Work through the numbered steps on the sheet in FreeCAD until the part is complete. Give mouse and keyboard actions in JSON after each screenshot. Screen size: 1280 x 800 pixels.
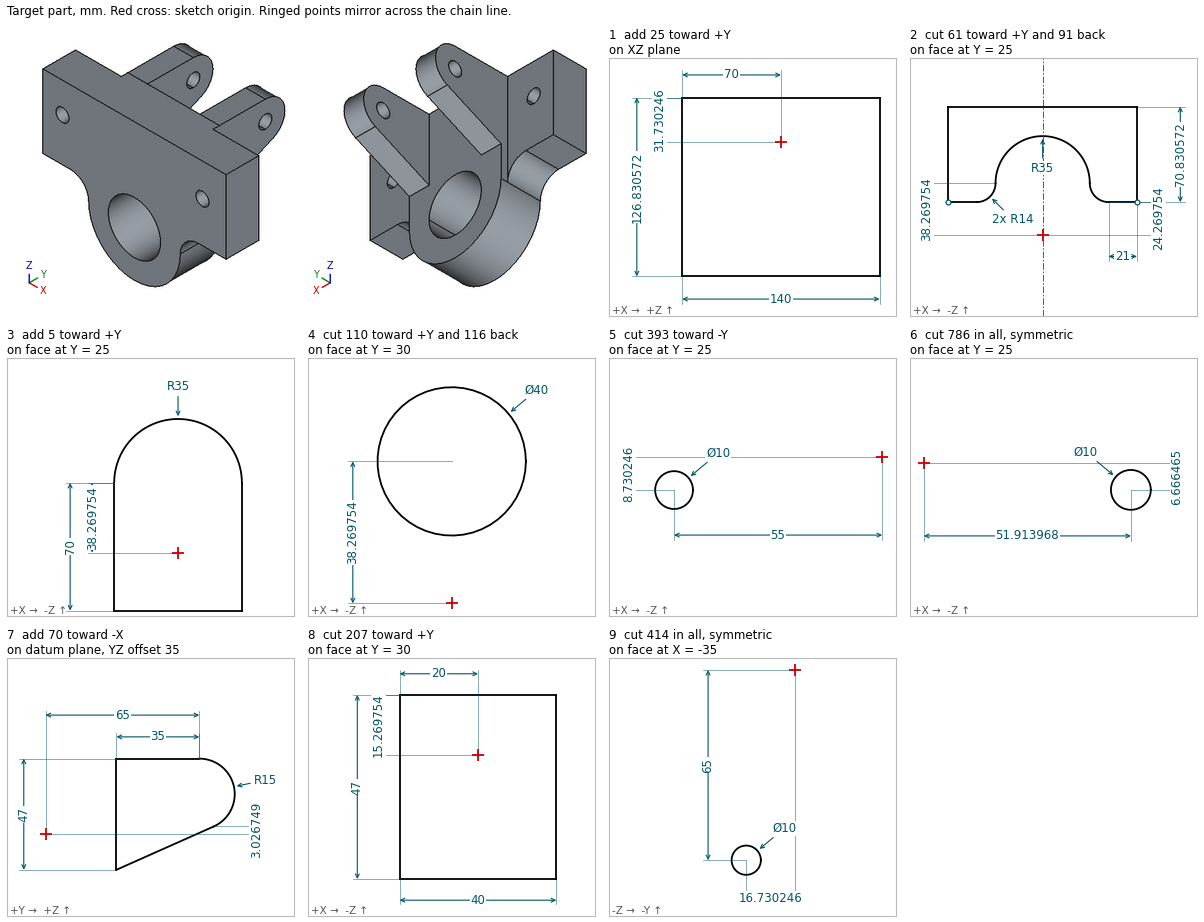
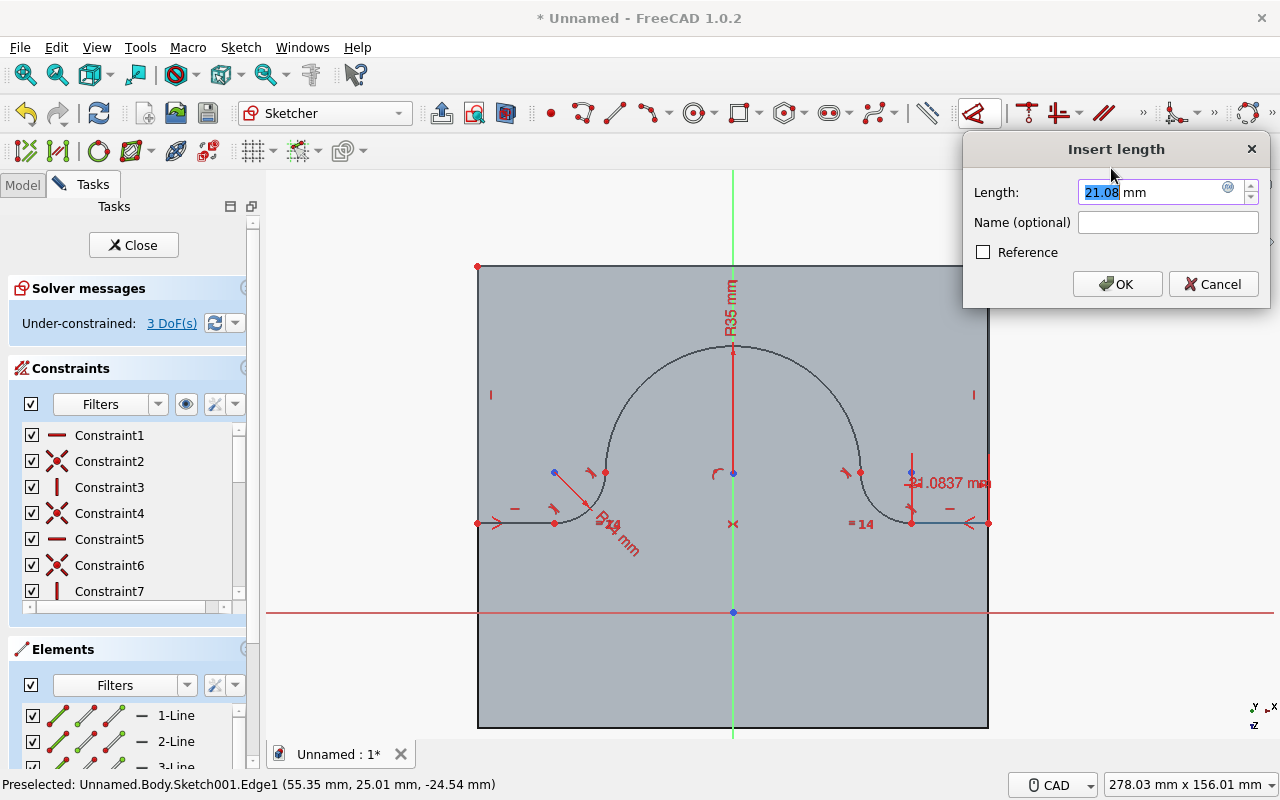
{"action": "type", "text": "21"}
{"action": "key", "text": "Return"}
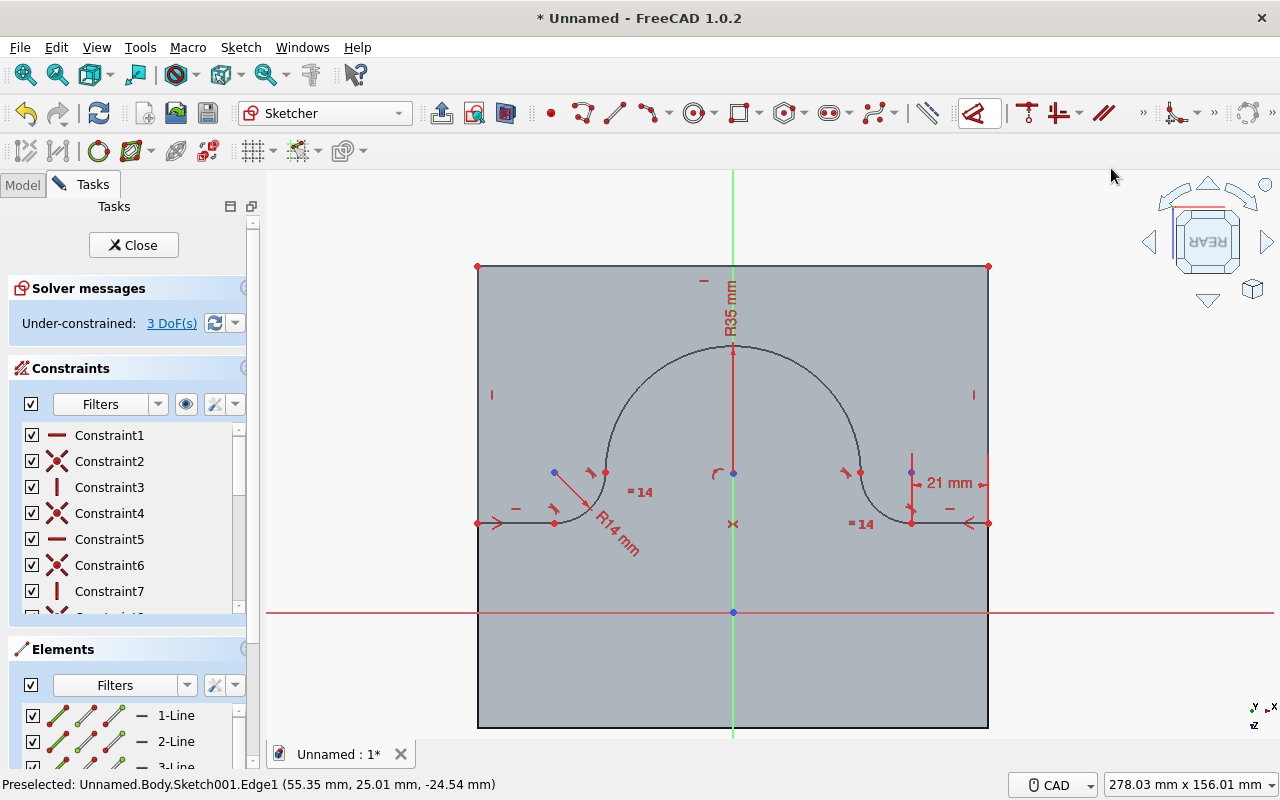
{"action": "left_click", "coordinate": [988, 446]}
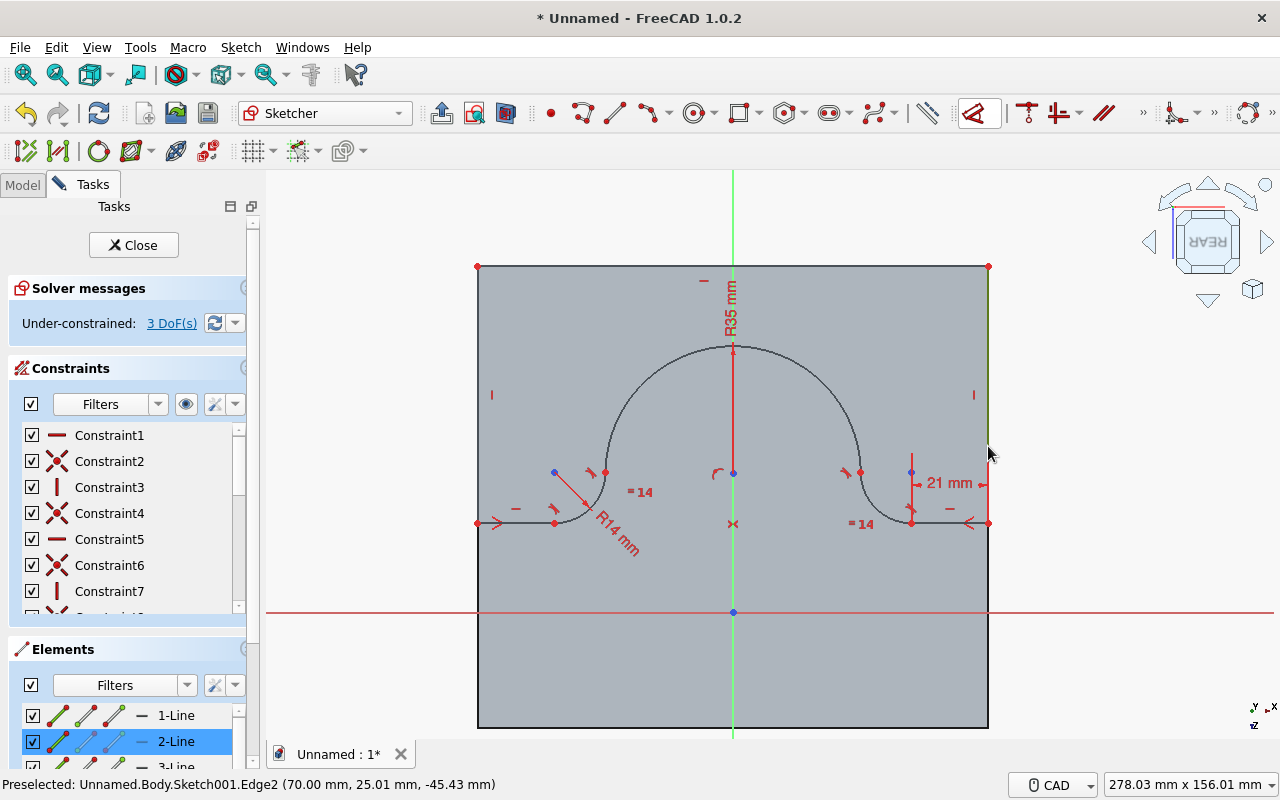
{"action": "key", "text": "i"}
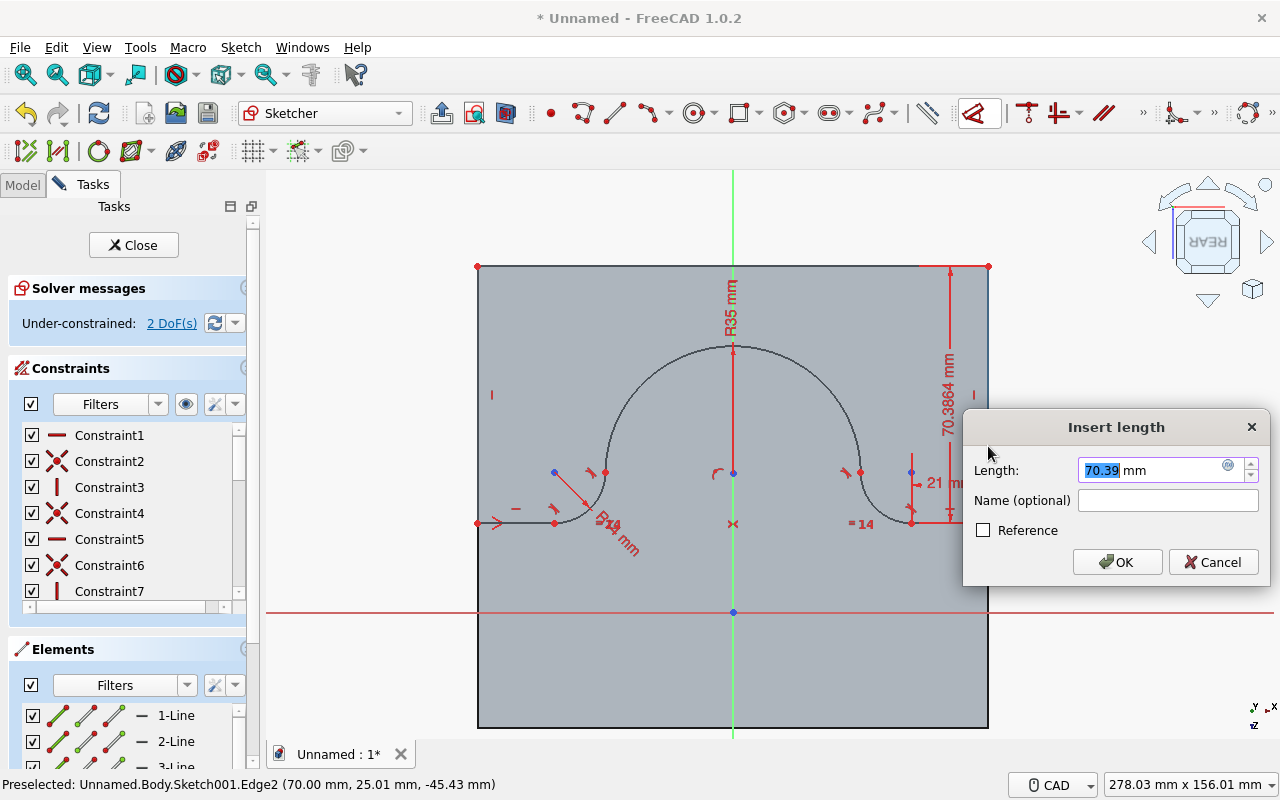
{"action": "type", "text": "70.830572"}
{"action": "key", "text": "Return"}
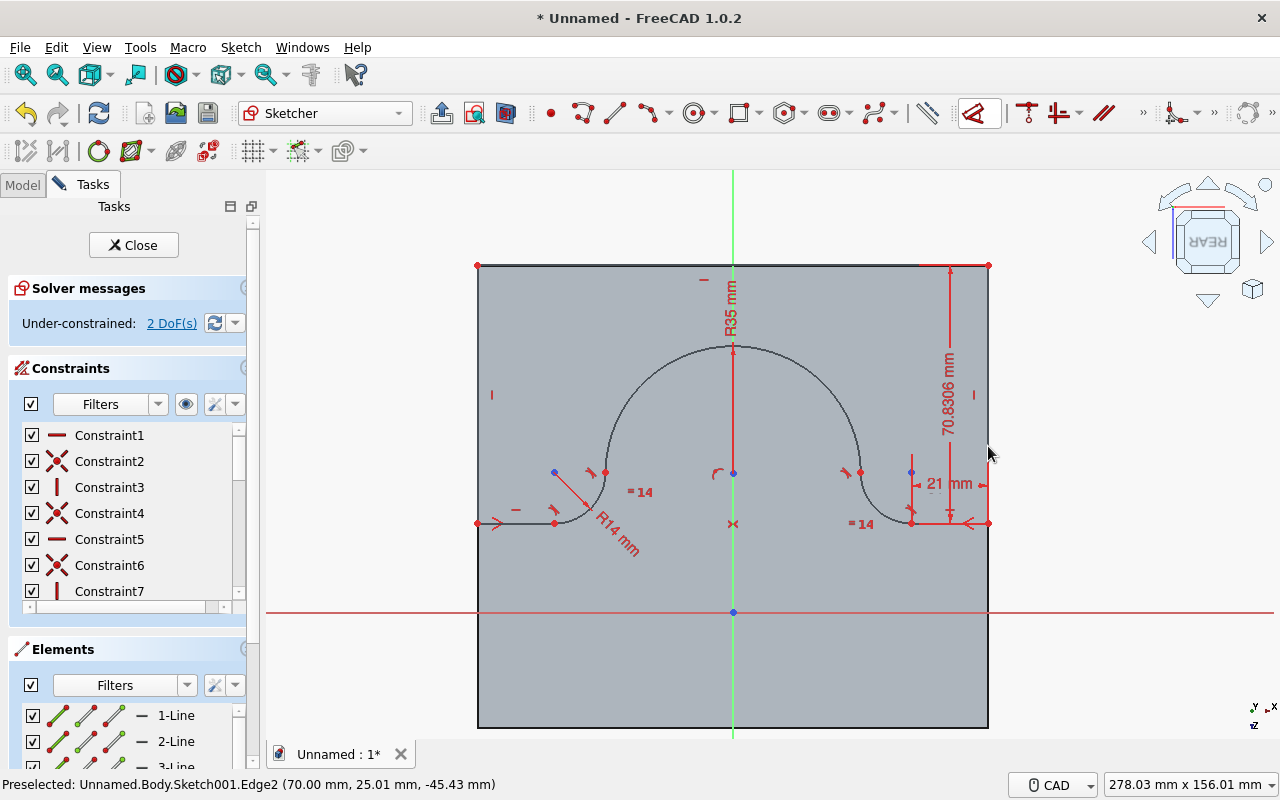
{"action": "left_click", "coordinate": [912, 524]}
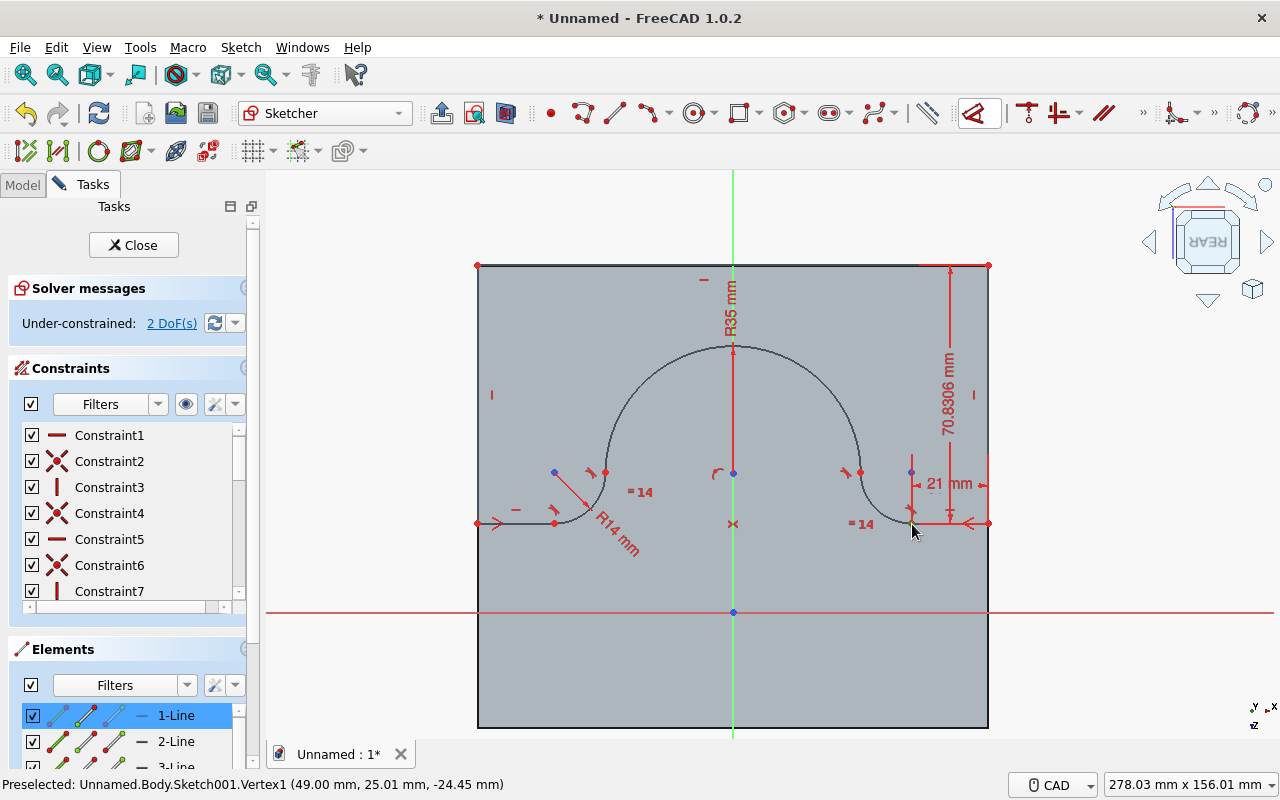
{"action": "key", "text": "i"}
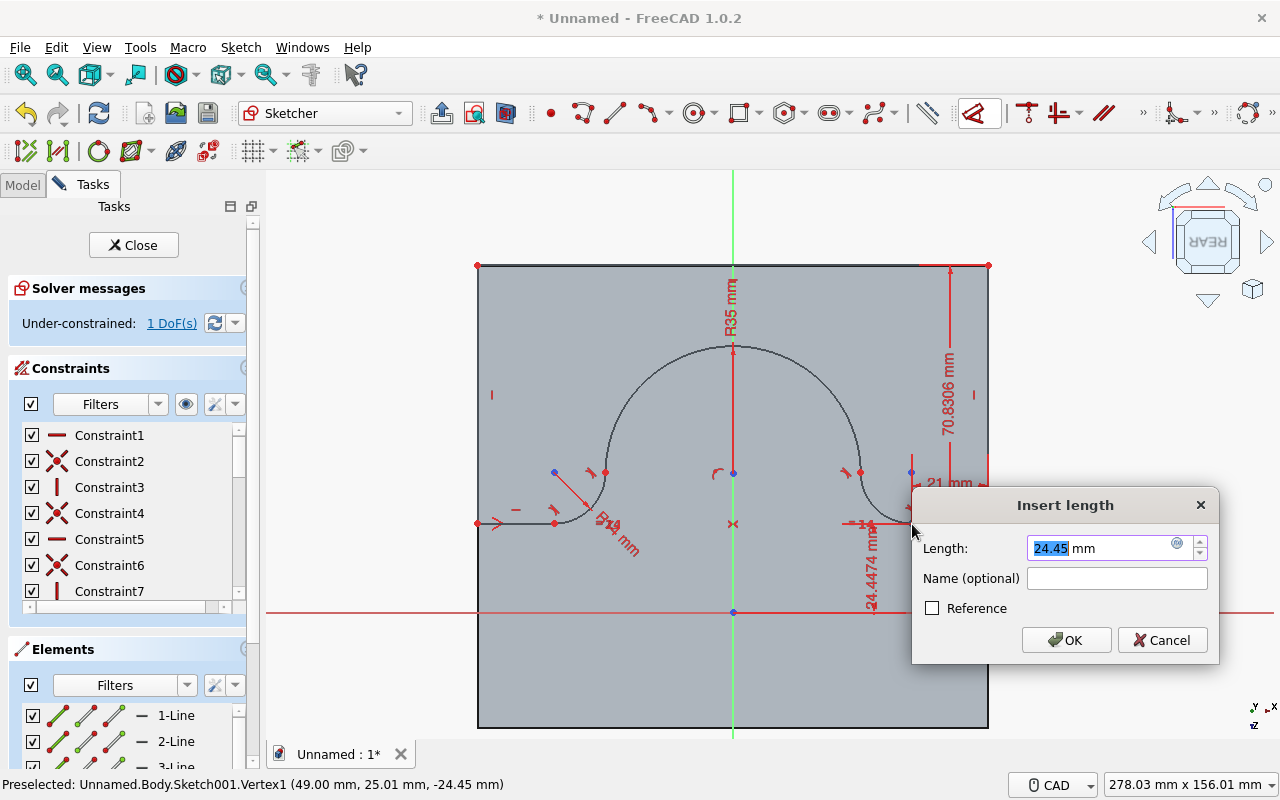
{"action": "type", "text": "24.269754"}
{"action": "key", "text": "Return"}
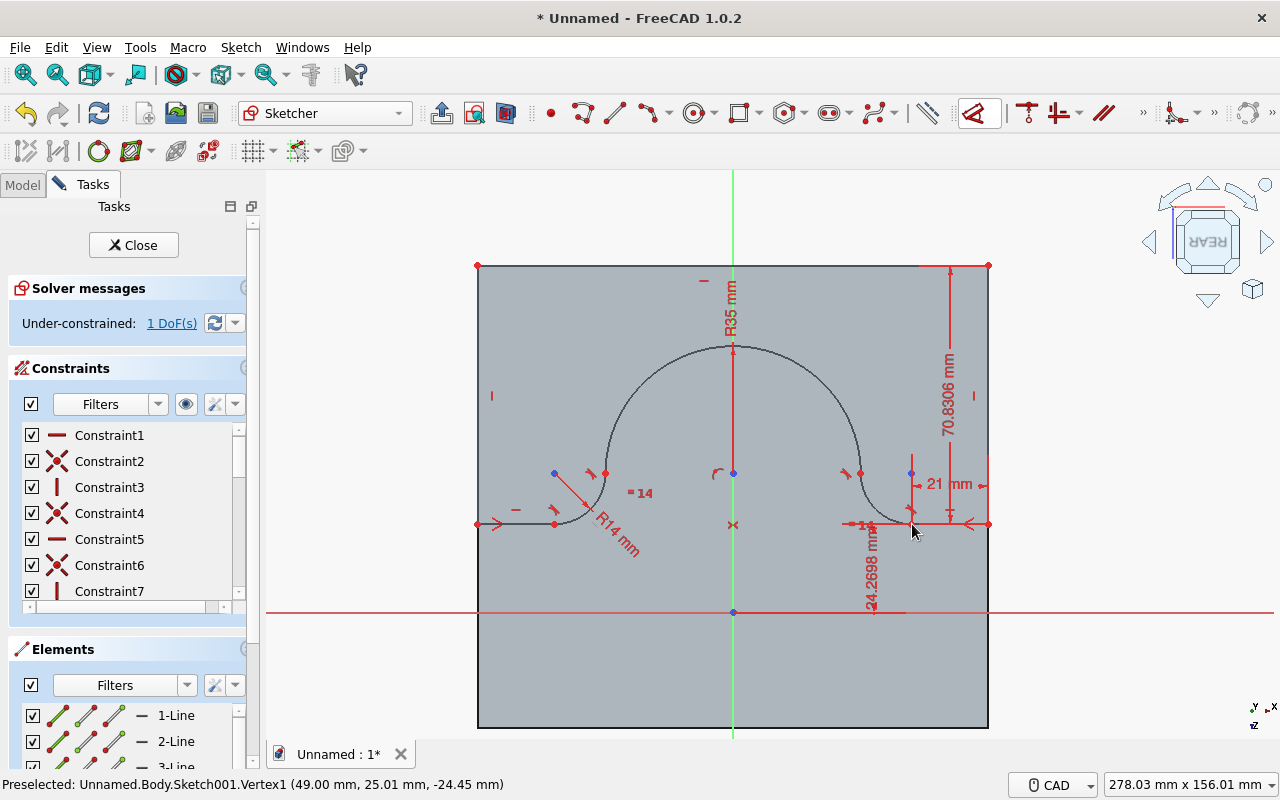
{"action": "left_click", "coordinate": [605, 473]}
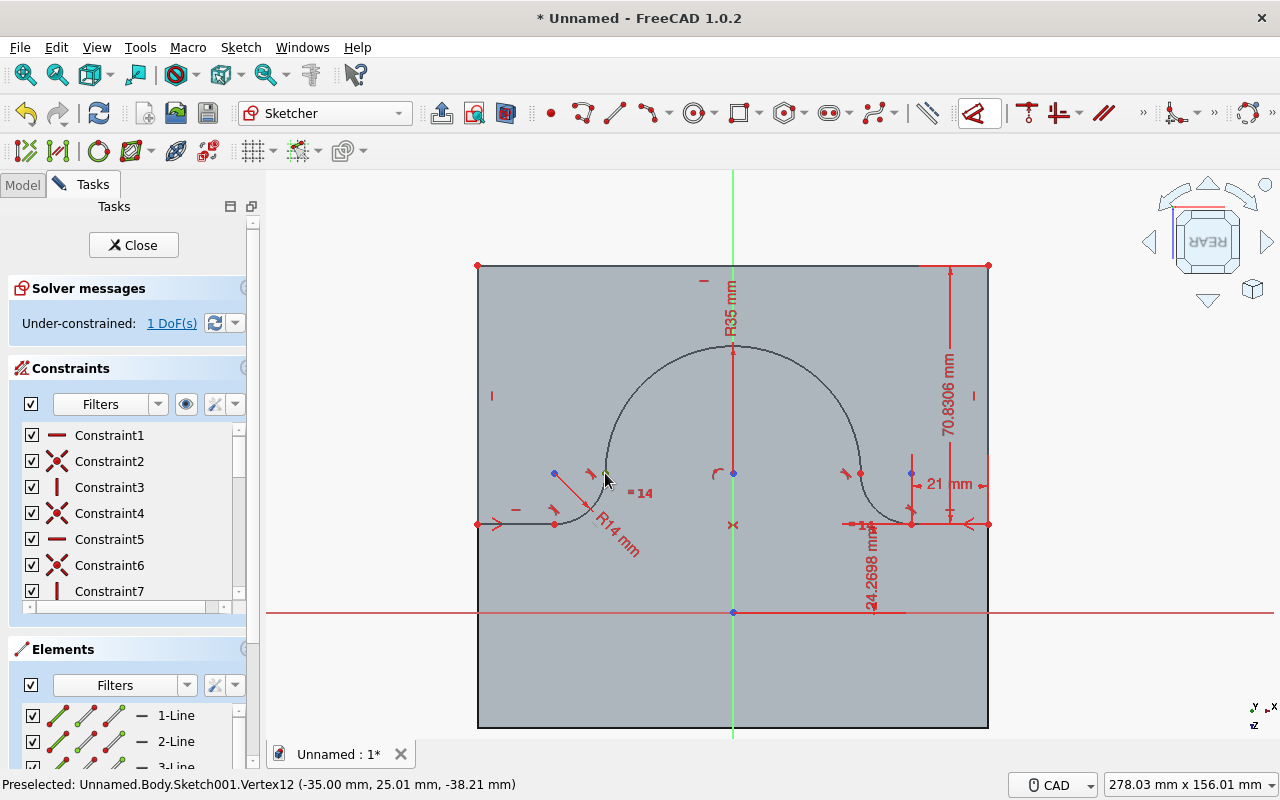
{"action": "left_click", "coordinate": [996, 114]}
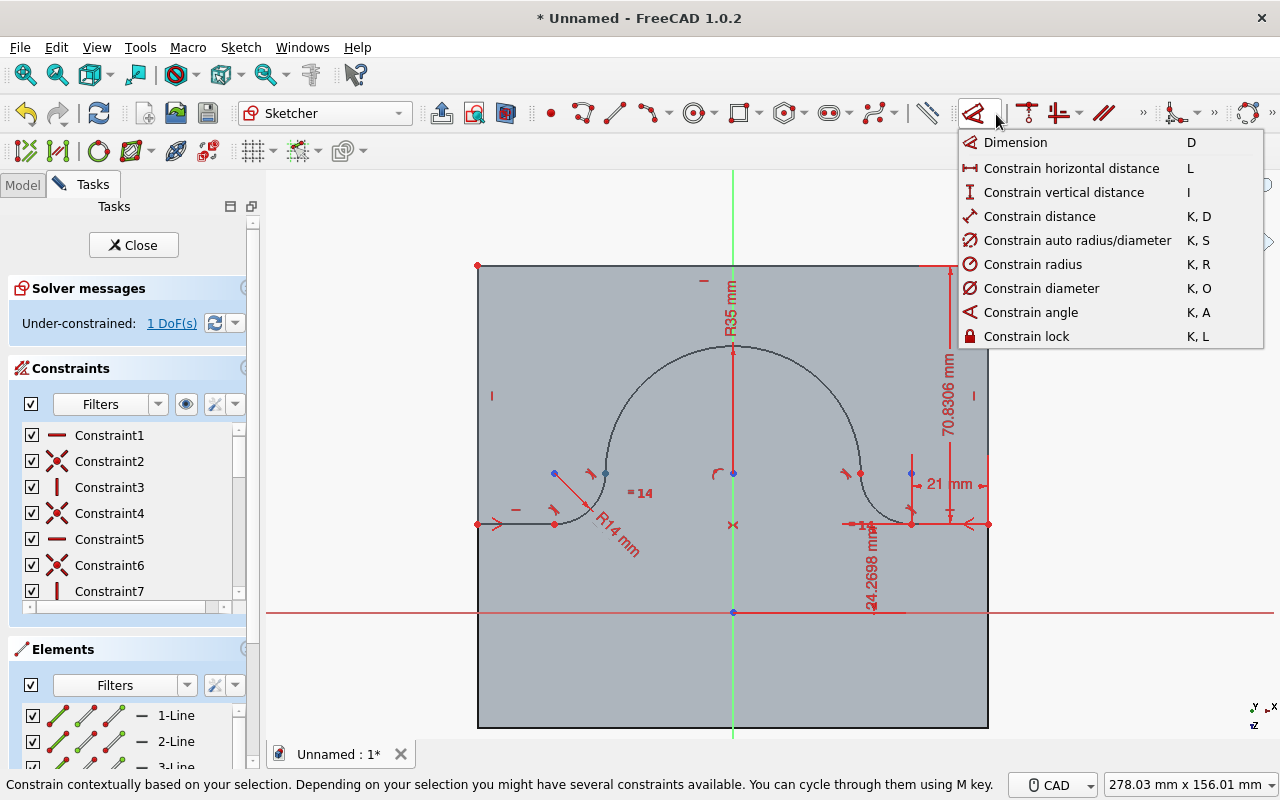
{"action": "left_click", "coordinate": [1111, 192]}